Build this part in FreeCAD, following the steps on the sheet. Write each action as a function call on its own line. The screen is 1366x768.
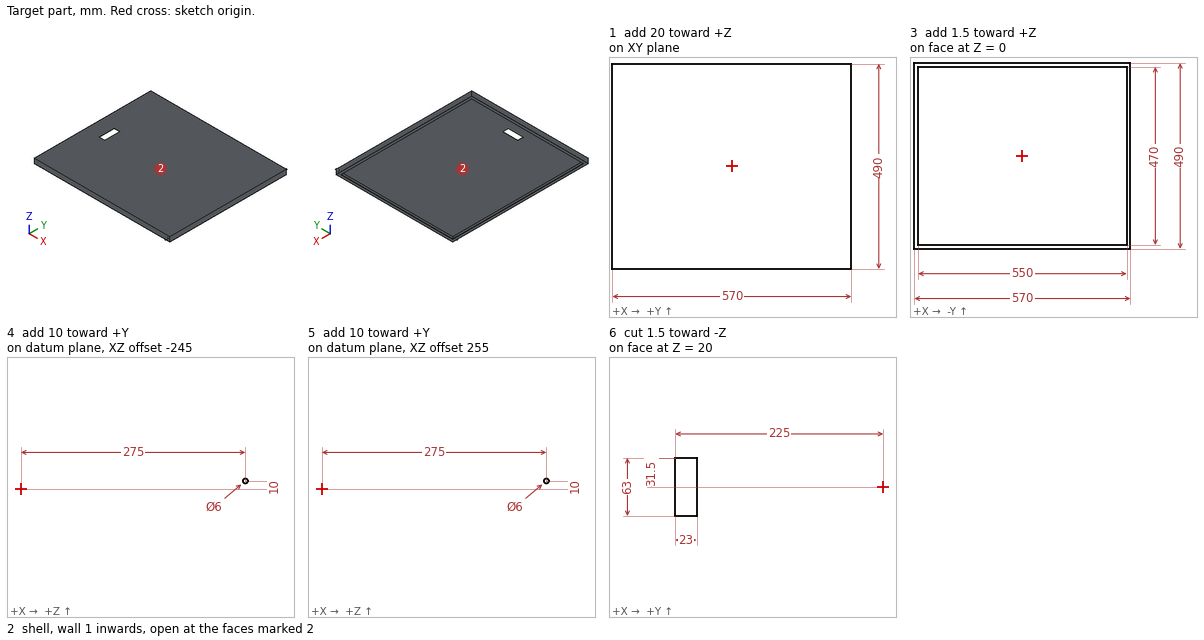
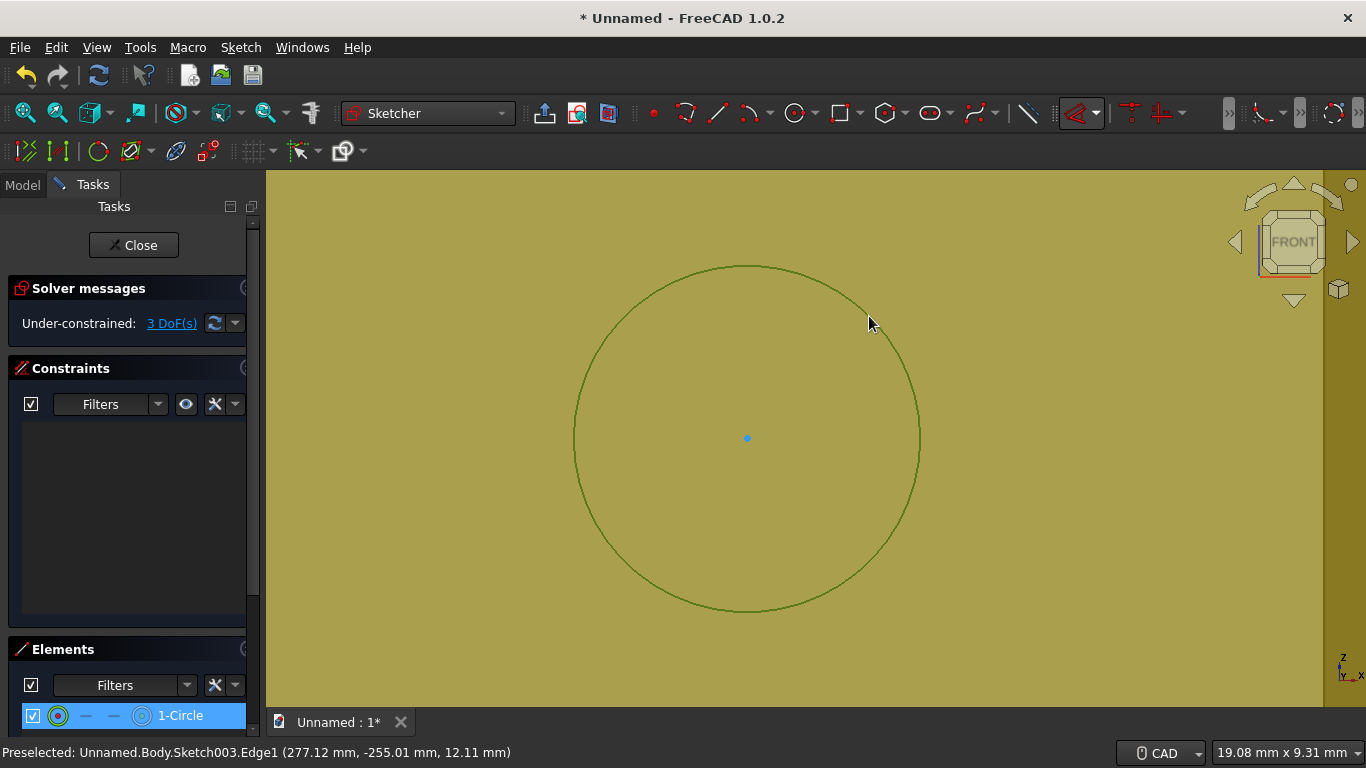
key(k)
key(o)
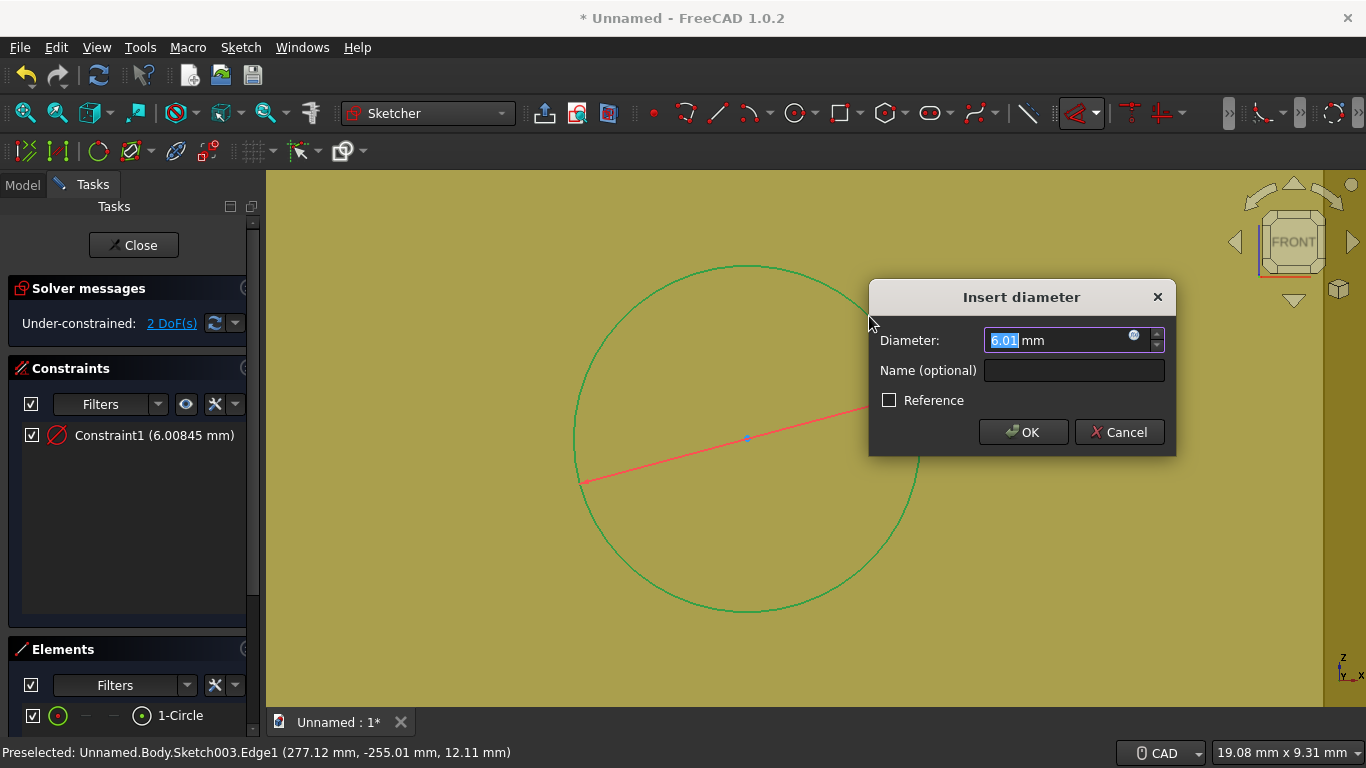
text(6)
key(Return)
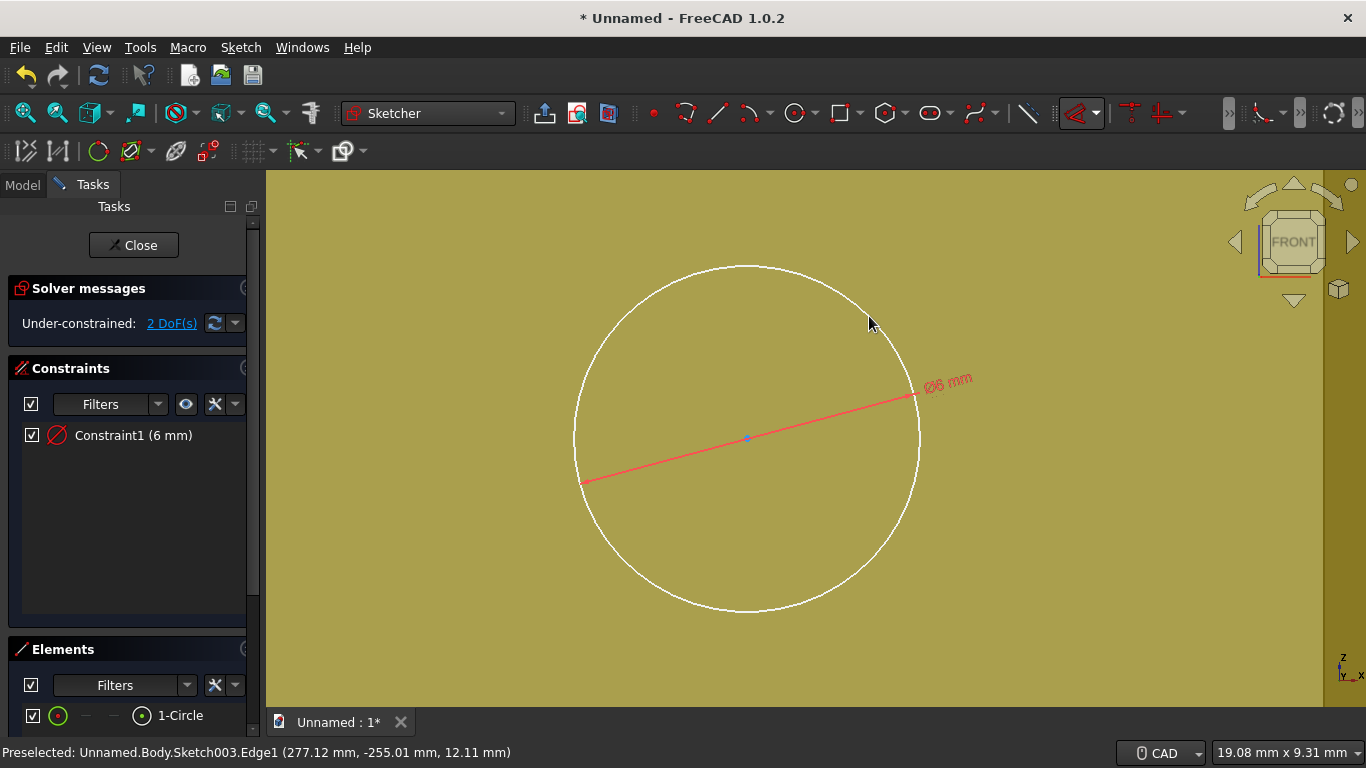
click(747, 439)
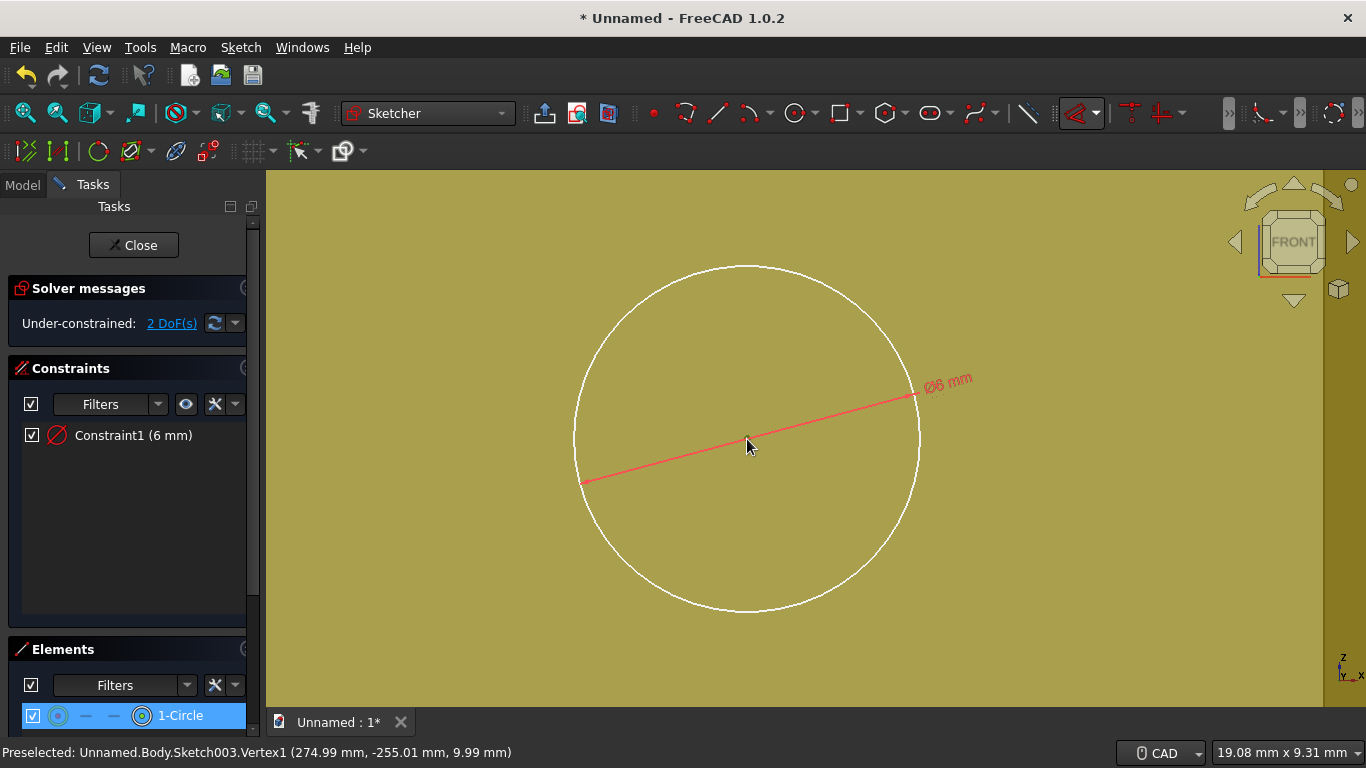
key(i)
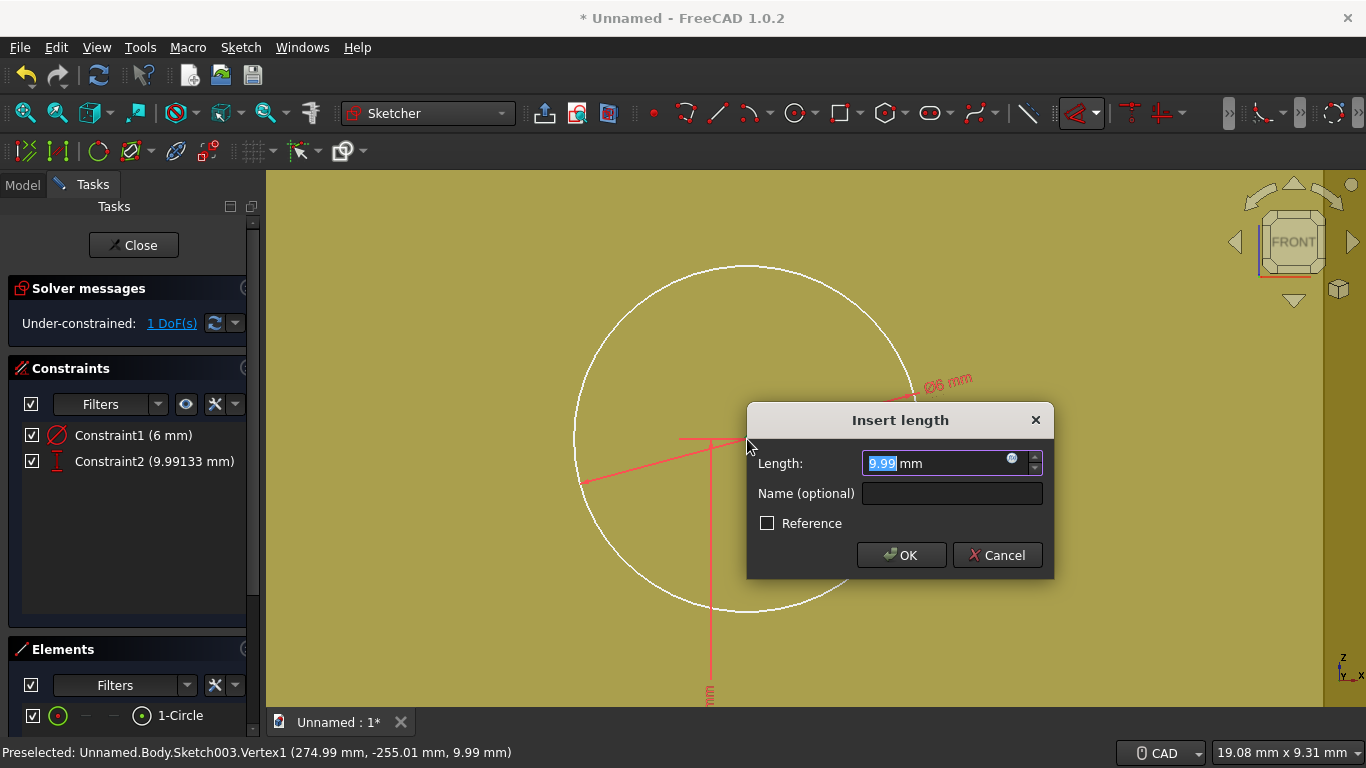
text(10)
key(Return)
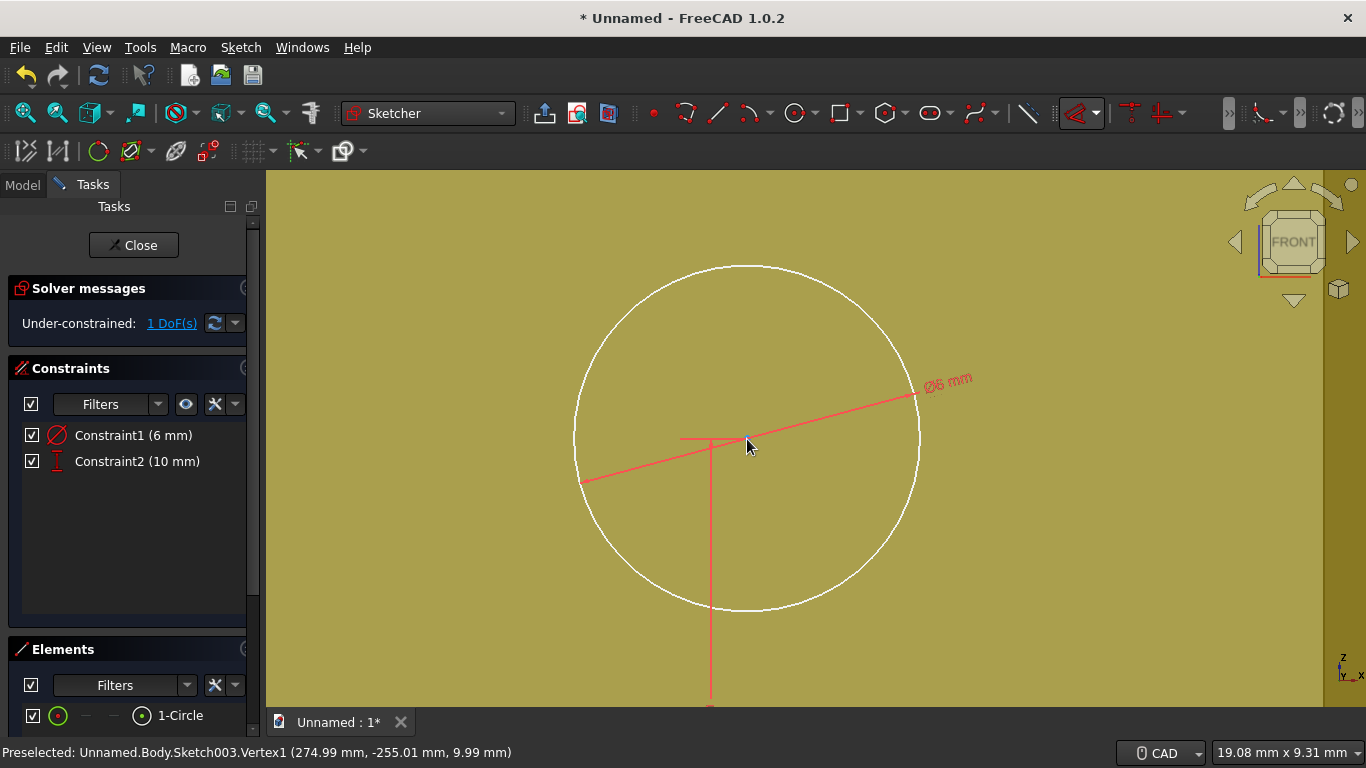
click(747, 438)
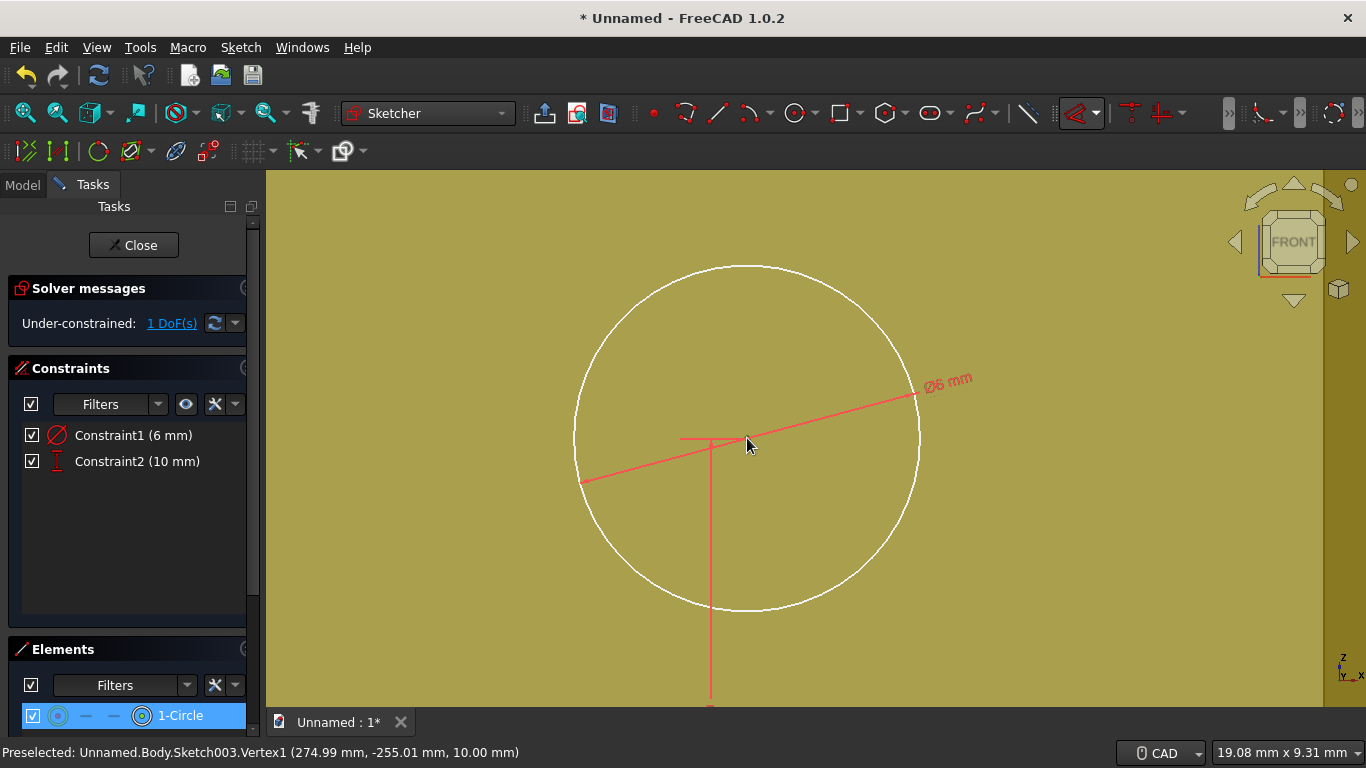
key(l)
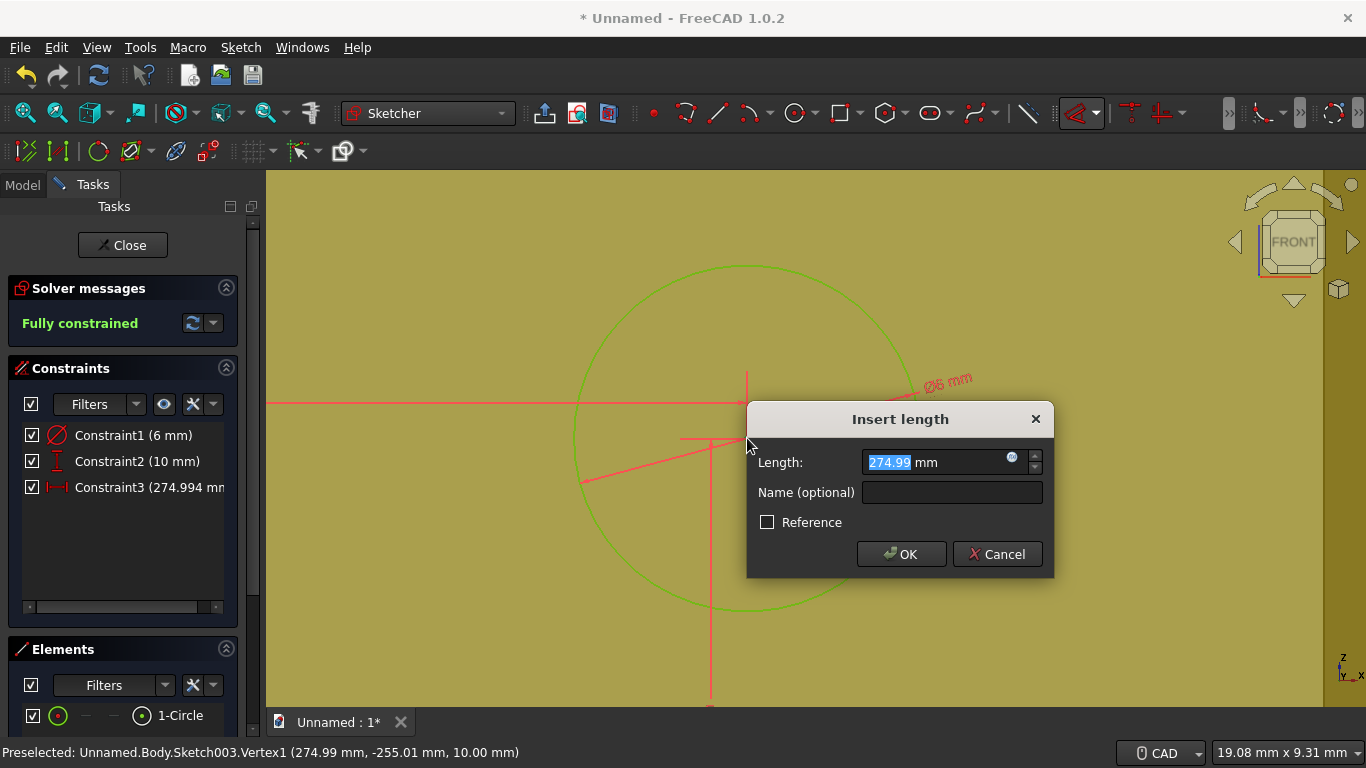
text(275)
key(Return)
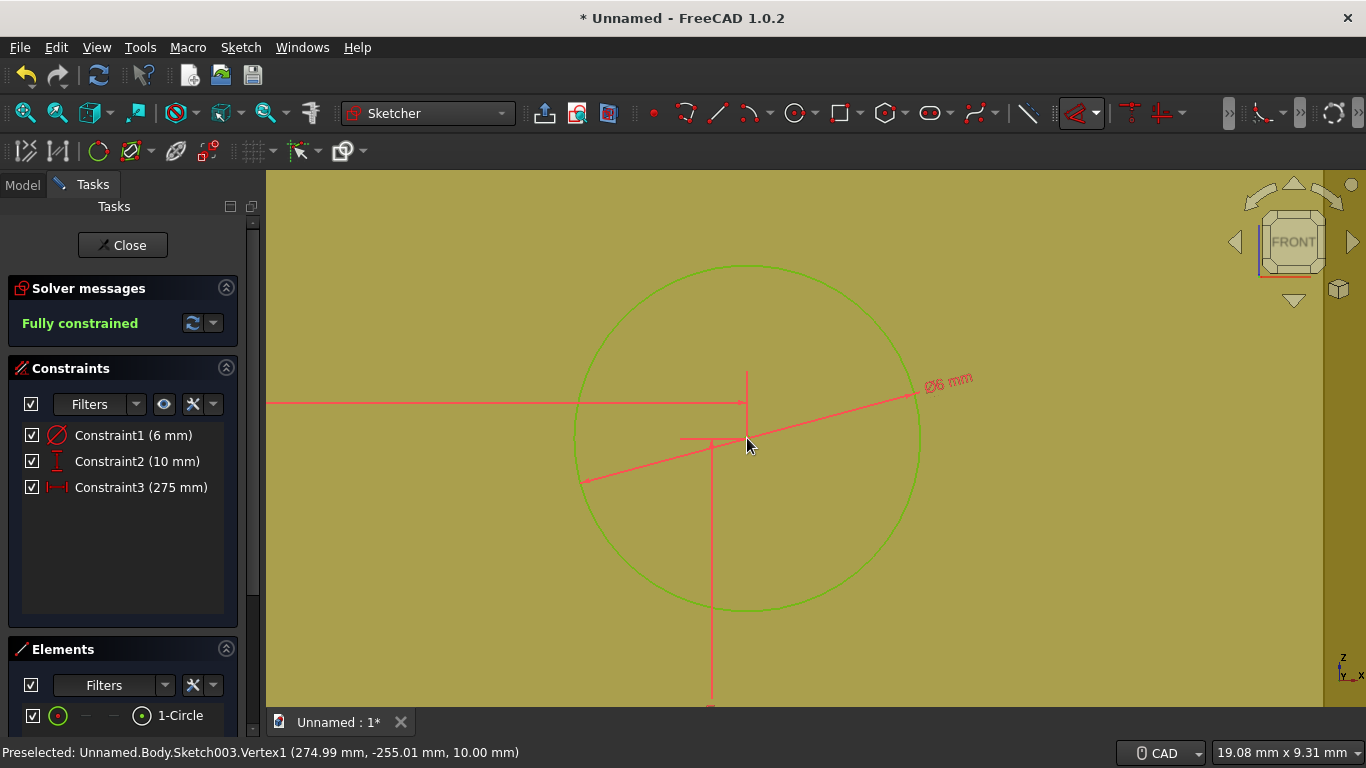
click(123, 245)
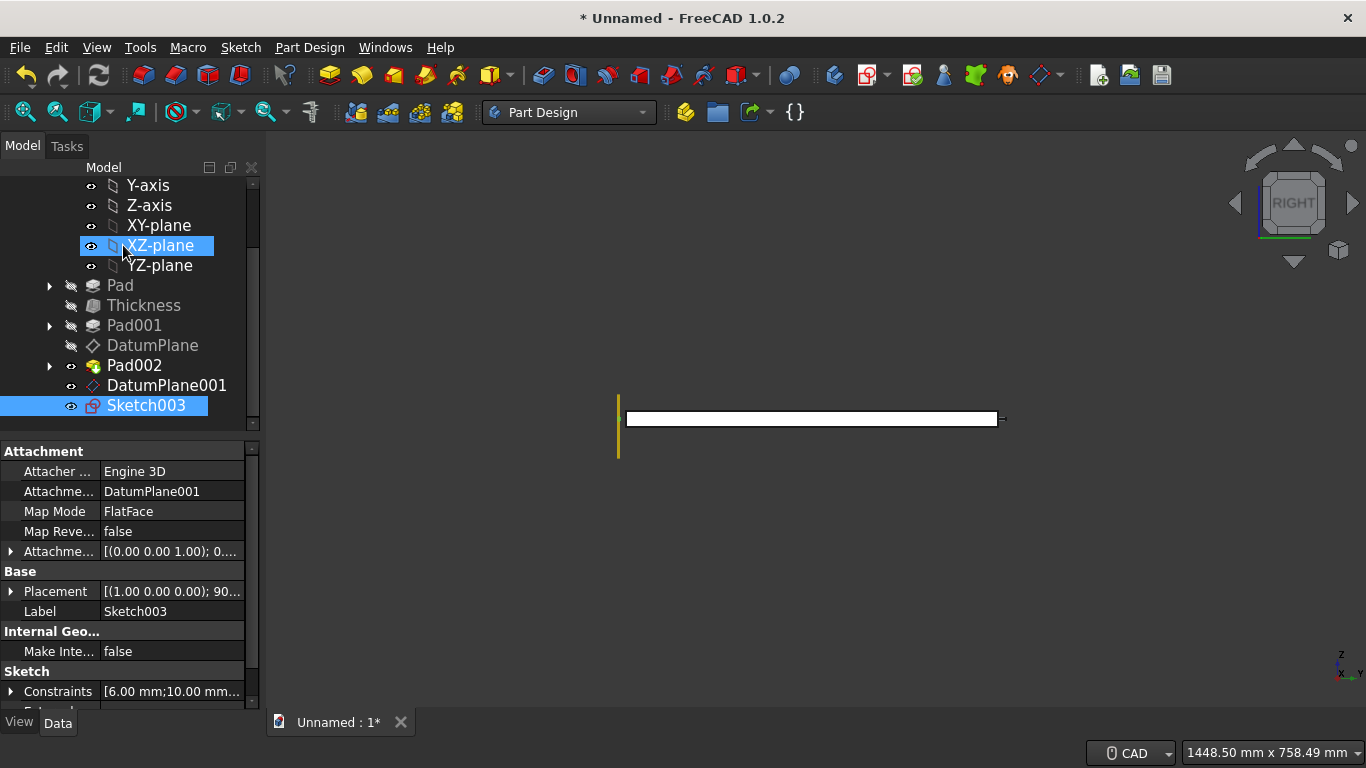
click(330, 76)